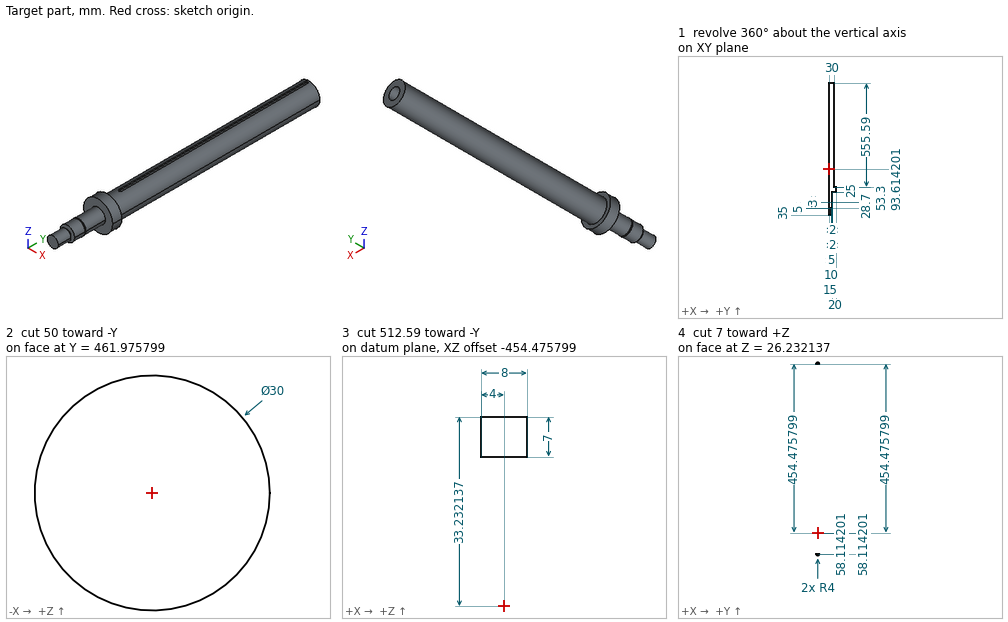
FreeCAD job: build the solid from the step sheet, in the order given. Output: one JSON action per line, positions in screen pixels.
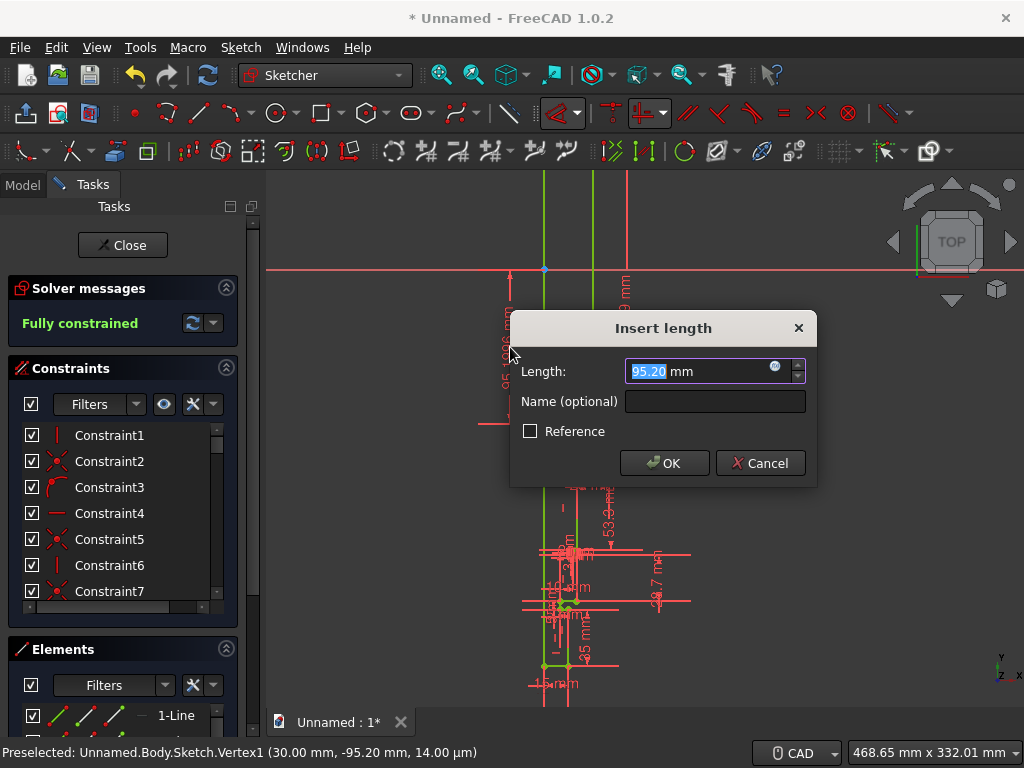
{"action": "type", "text": "93.614201"}
{"action": "key", "text": "Return"}
{"action": "key", "text": "Escape"}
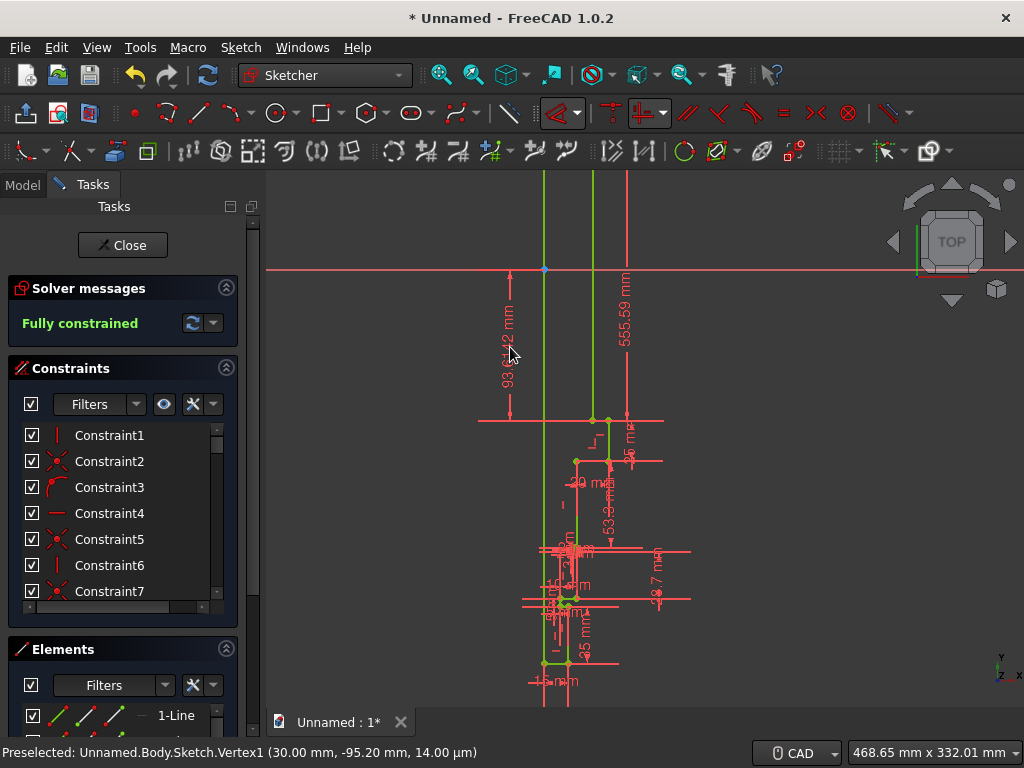
{"action": "left_click", "coordinate": [123, 245]}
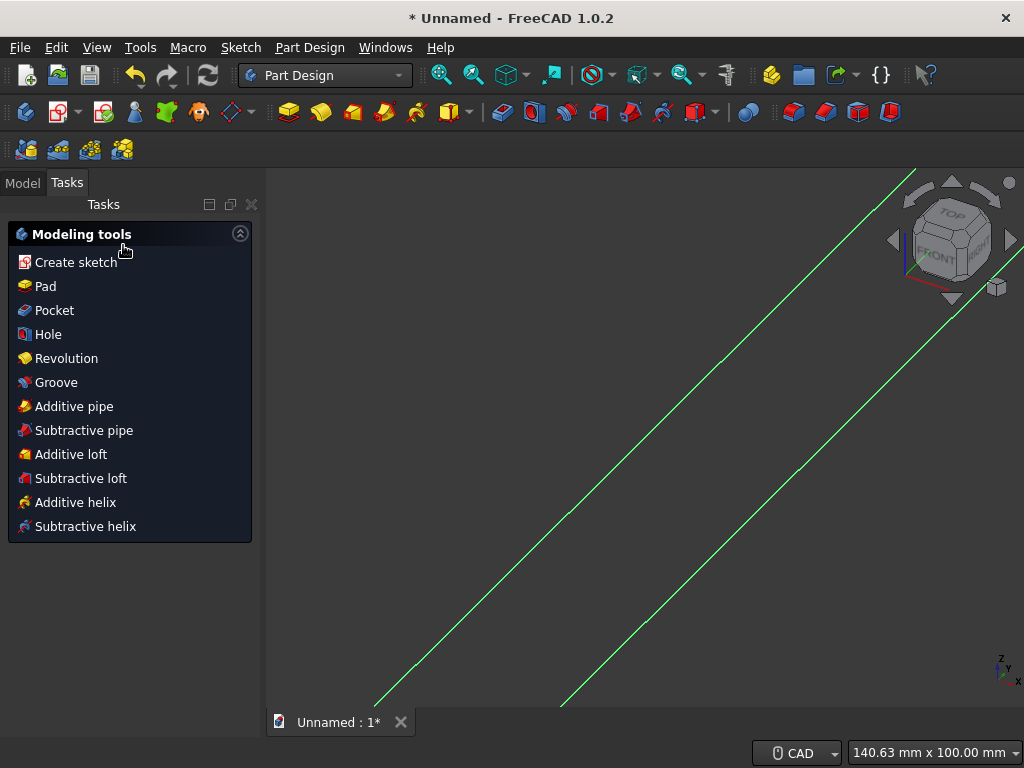
{"action": "left_click", "coordinate": [322, 112]}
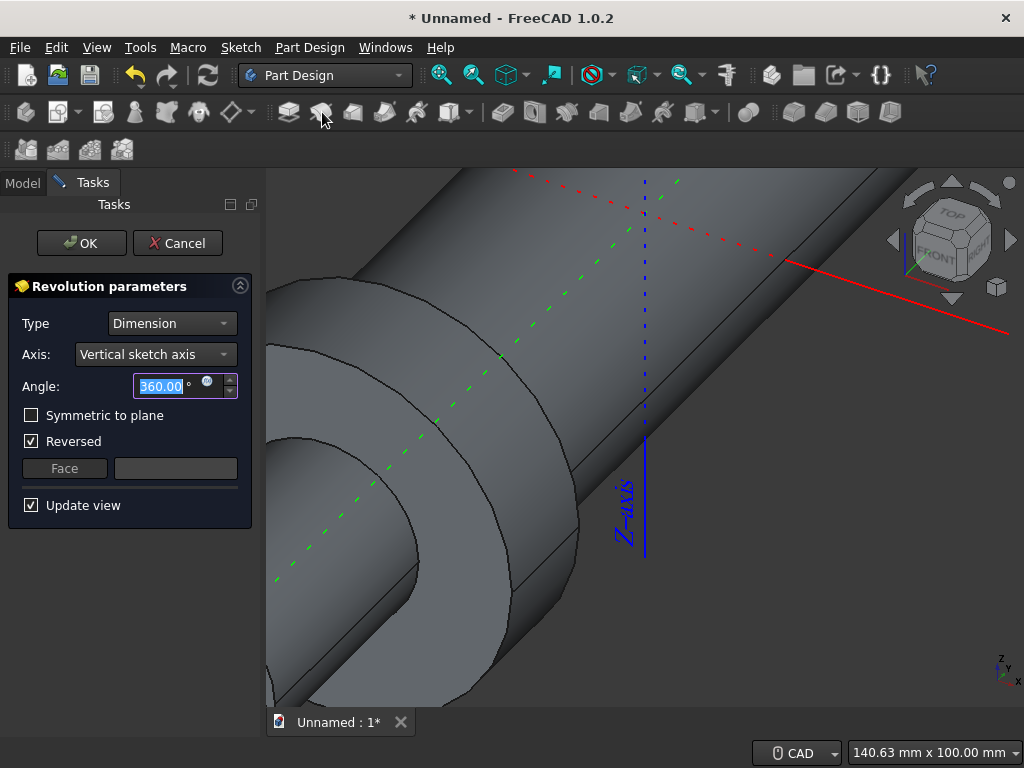
{"action": "left_click", "coordinate": [82, 243]}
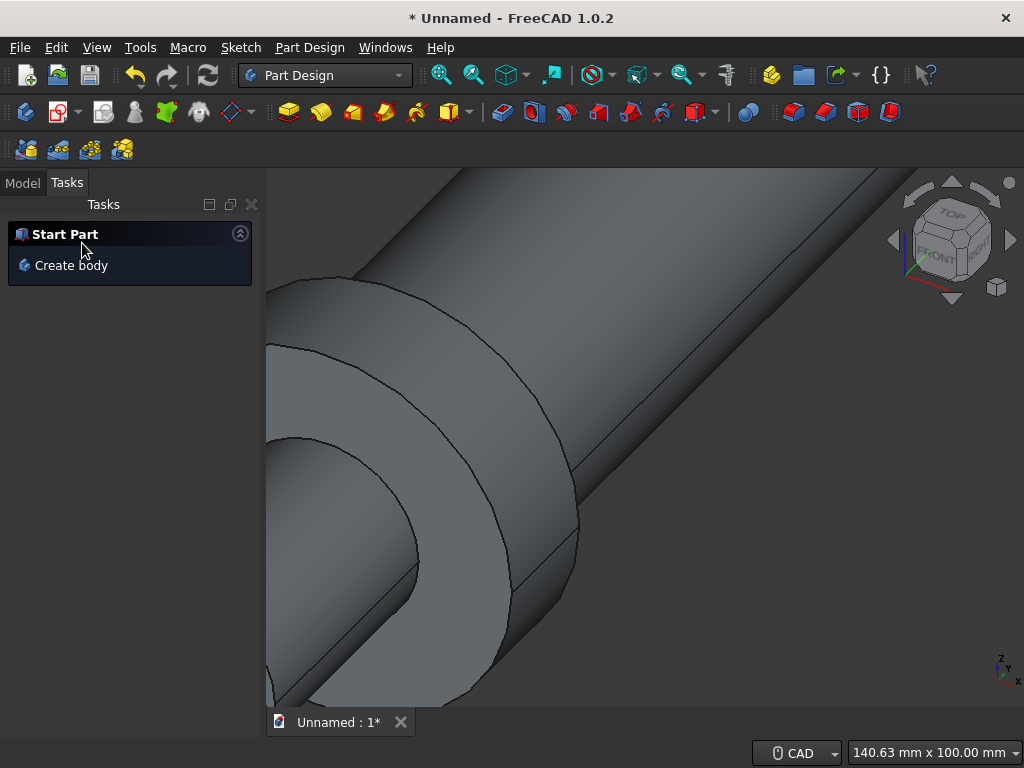
{"action": "left_click", "coordinate": [442, 76]}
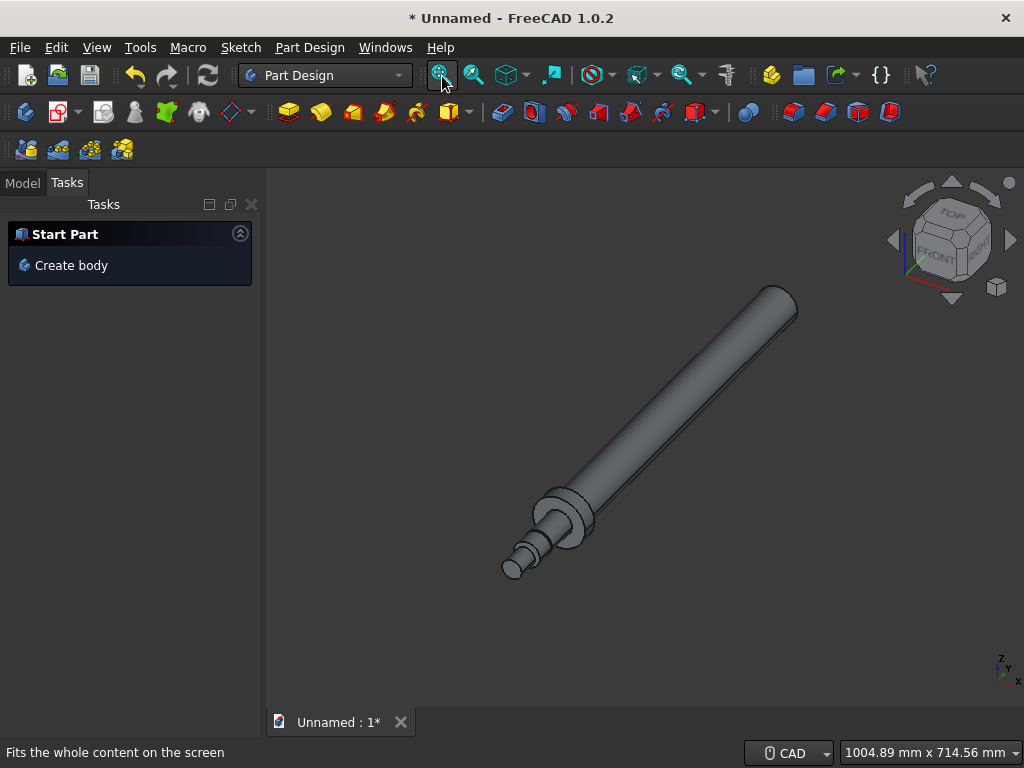
{"action": "key", "text": "4"}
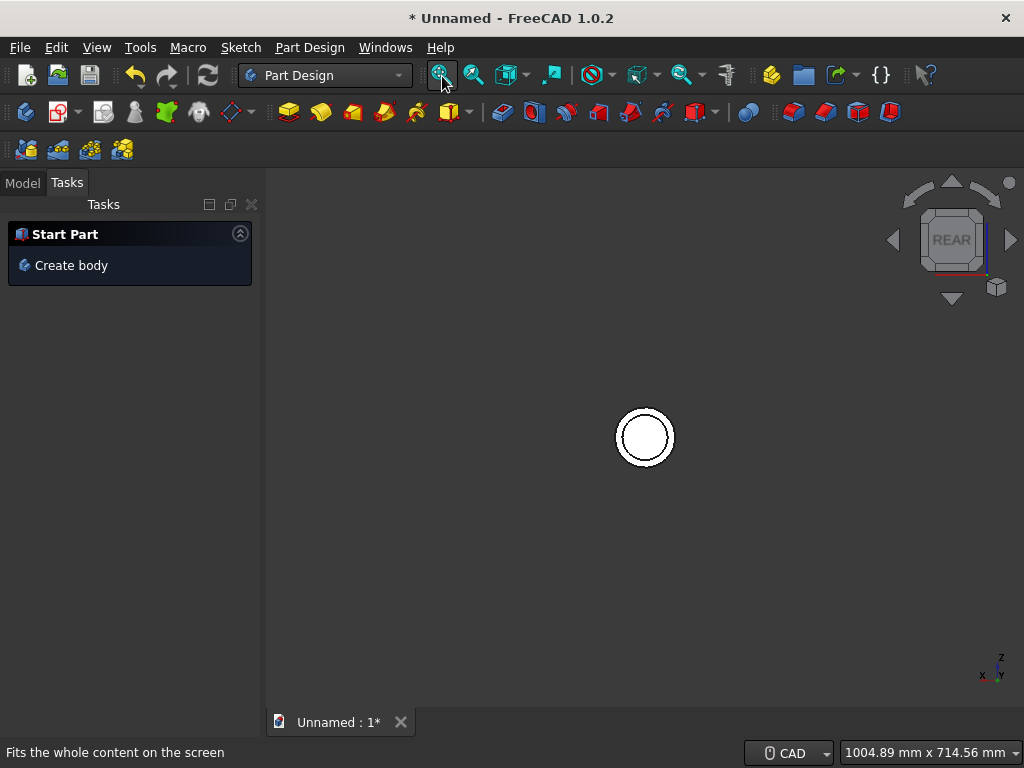
{"action": "left_click", "coordinate": [442, 76]}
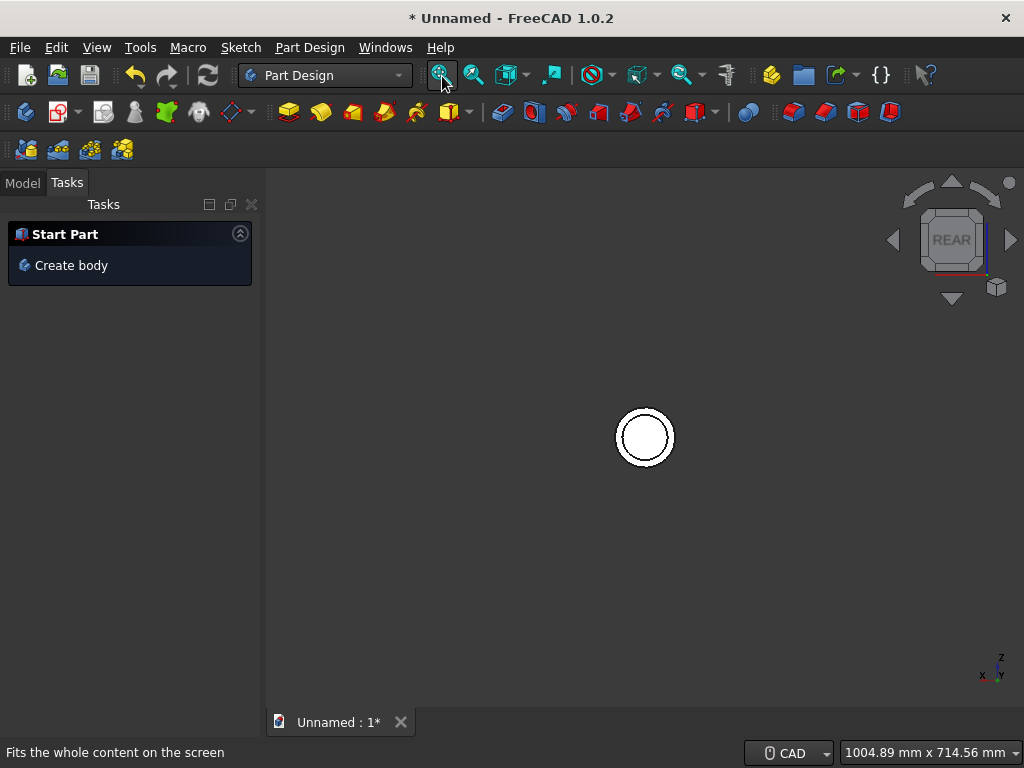
{"action": "left_click", "coordinate": [645, 437]}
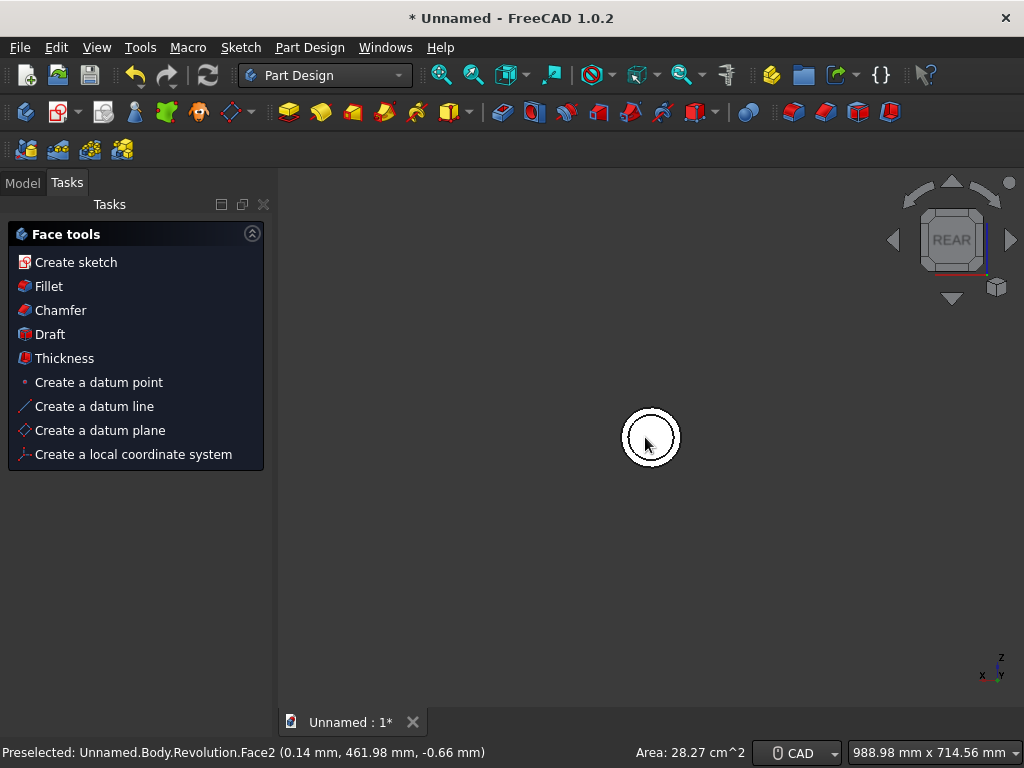
{"action": "left_click", "coordinate": [58, 112]}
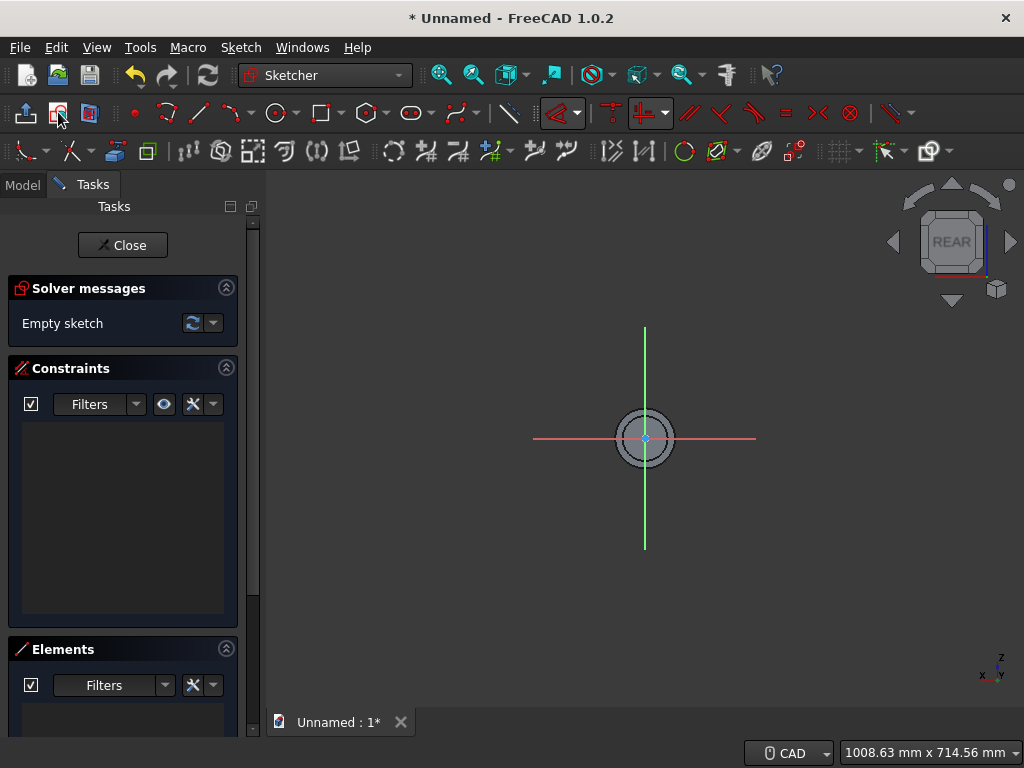
{"action": "scroll", "coordinate": [650, 439], "scroll_direction": "up", "scroll_amount": 14}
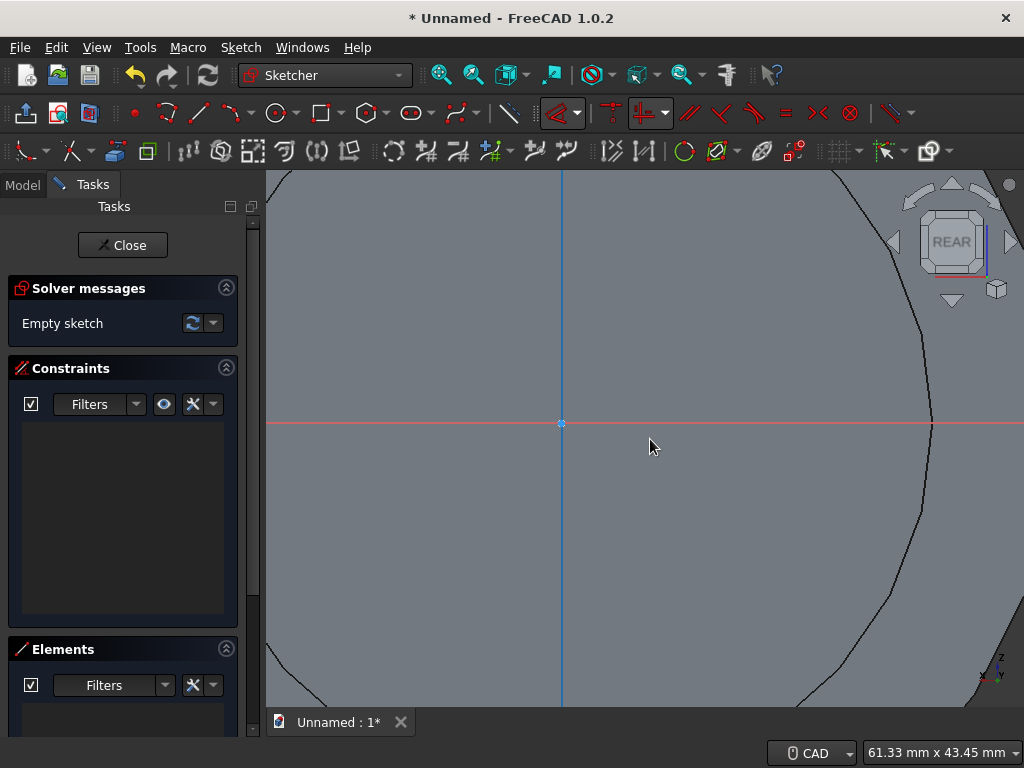
{"action": "key", "text": "g c"}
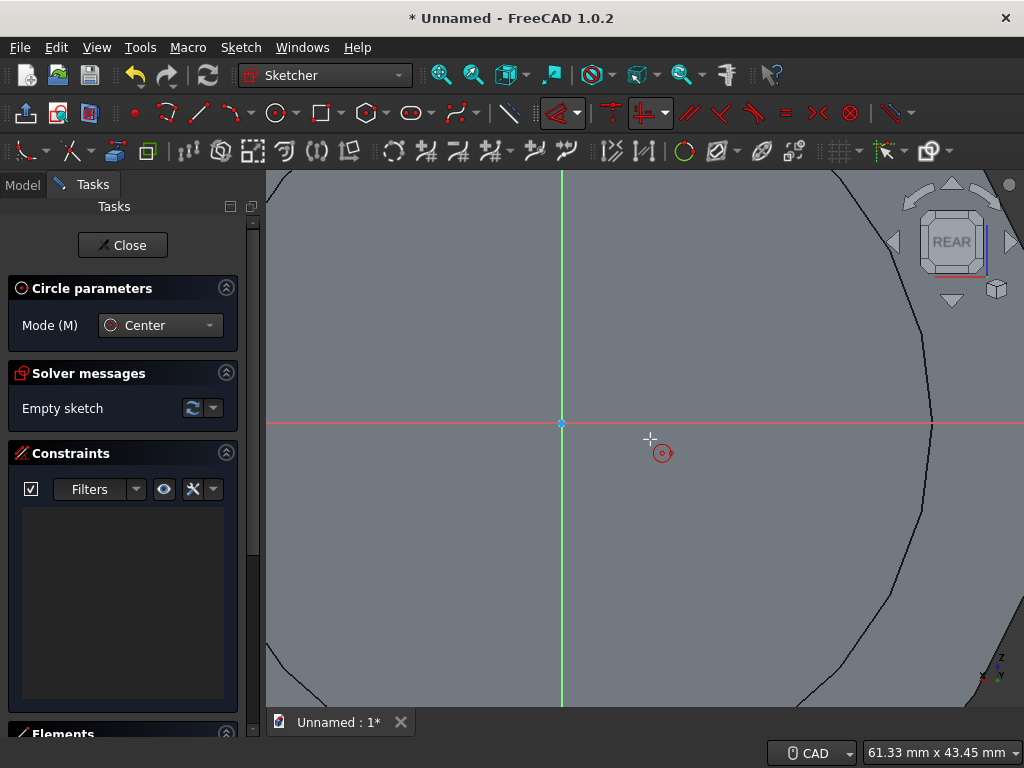
{"action": "left_click", "coordinate": [562, 423]}
{"action": "mouse_move", "coordinate": [693, 292]}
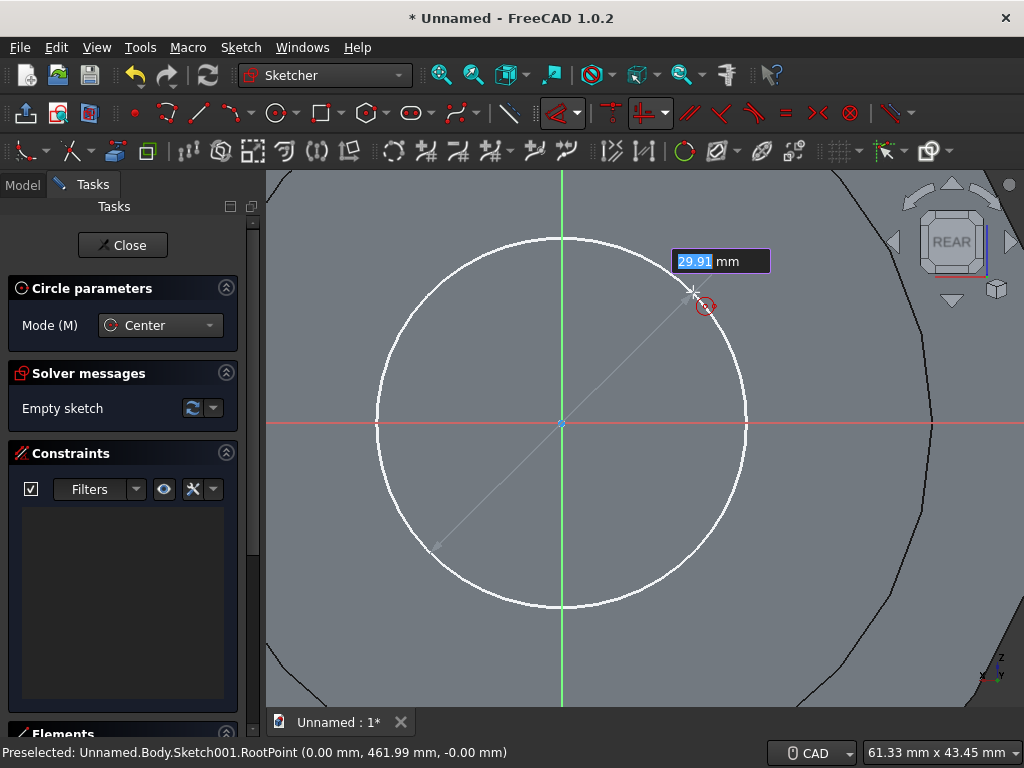
{"action": "type", "text": "30"}
{"action": "key", "text": "Return"}
{"action": "key", "text": "Escape"}